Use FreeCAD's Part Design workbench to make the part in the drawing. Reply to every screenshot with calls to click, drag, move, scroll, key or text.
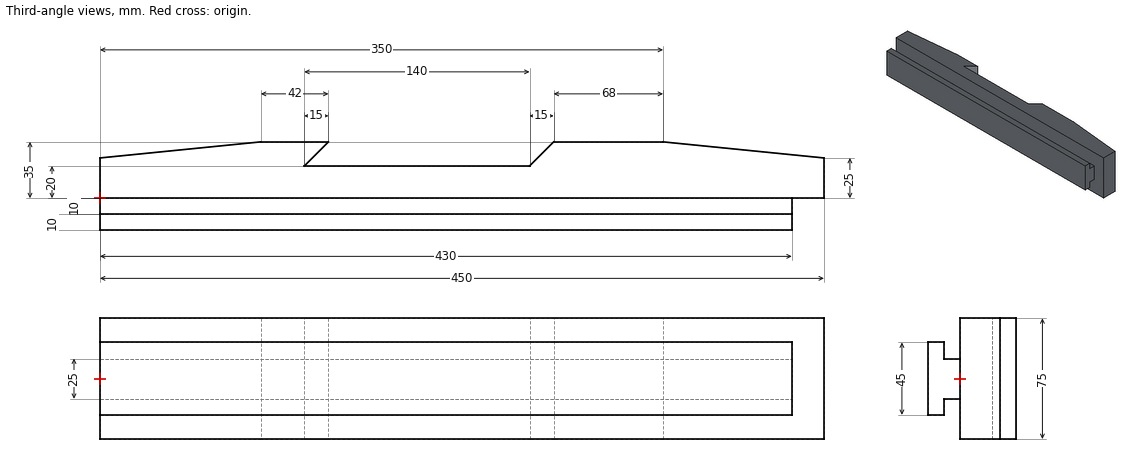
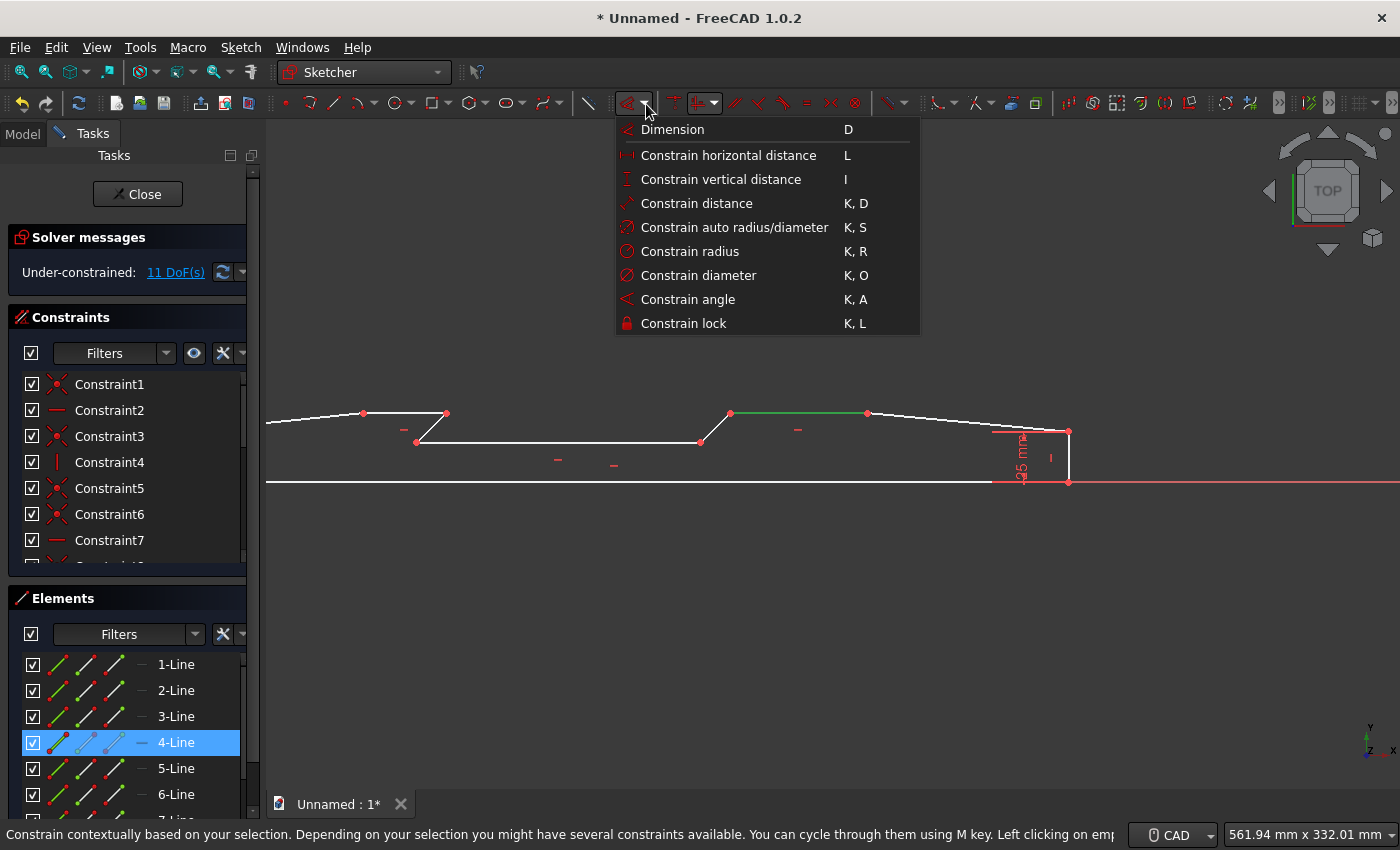
click(768, 155)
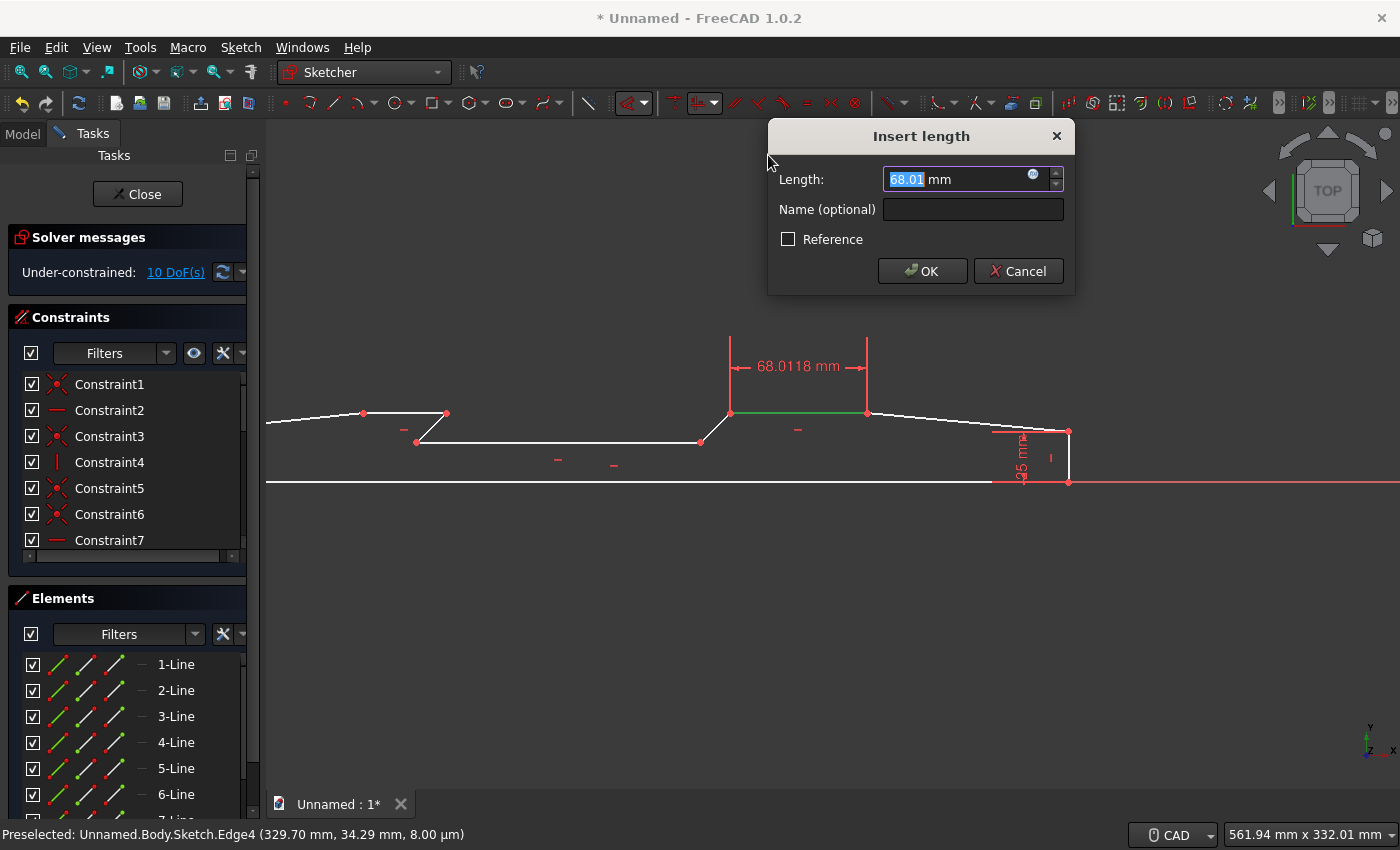
text(68)
key(Return)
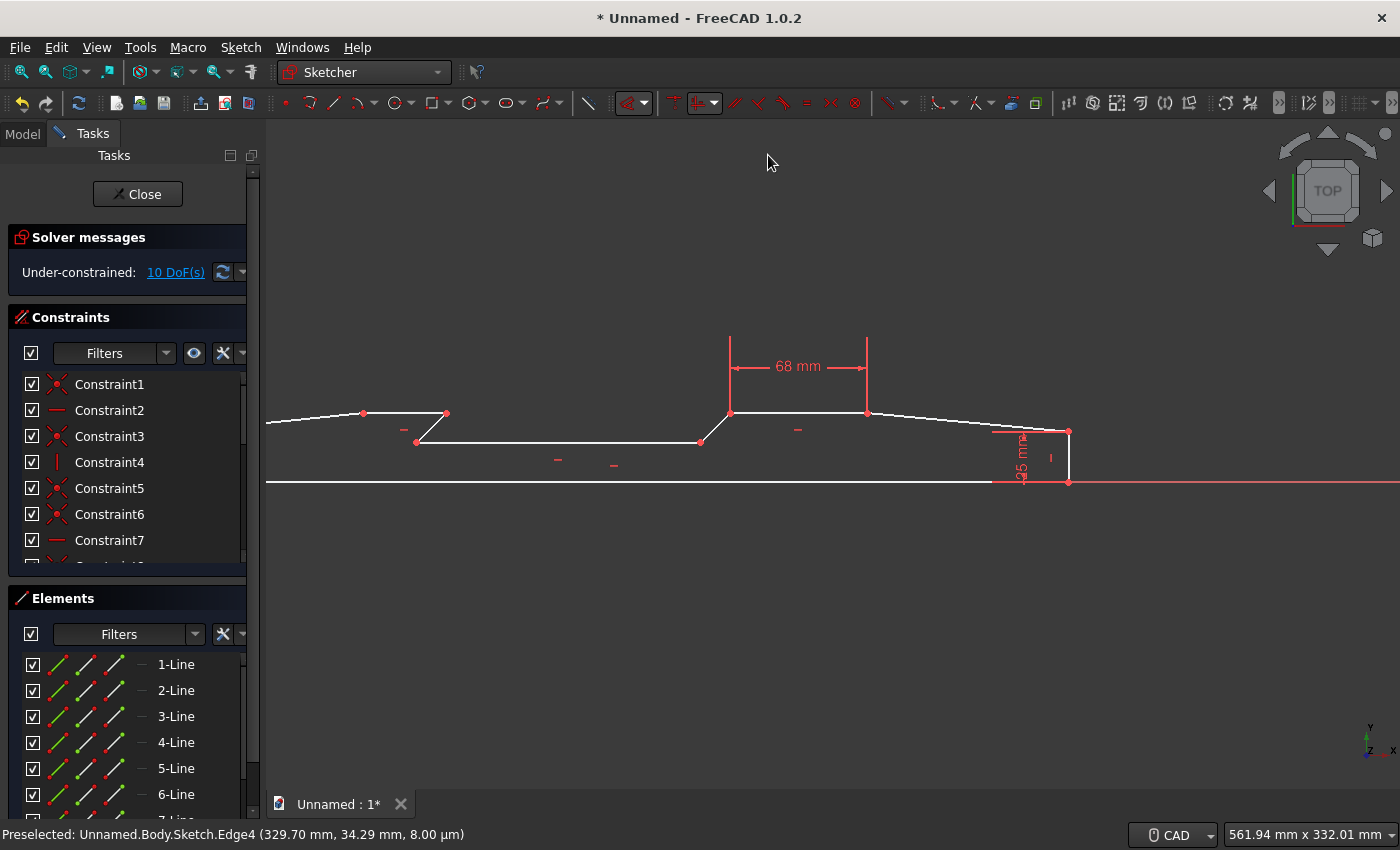
click(421, 413)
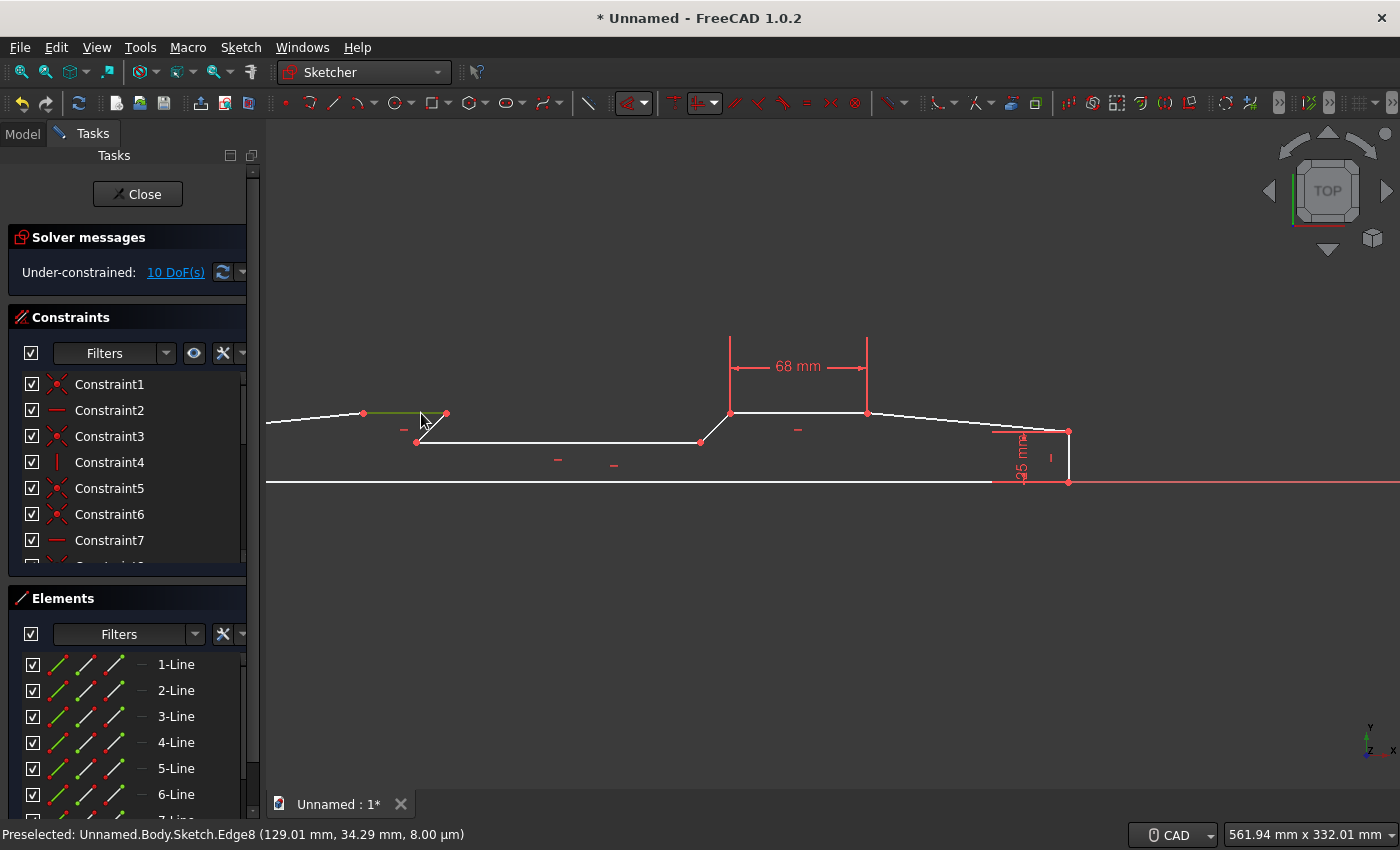
key(l)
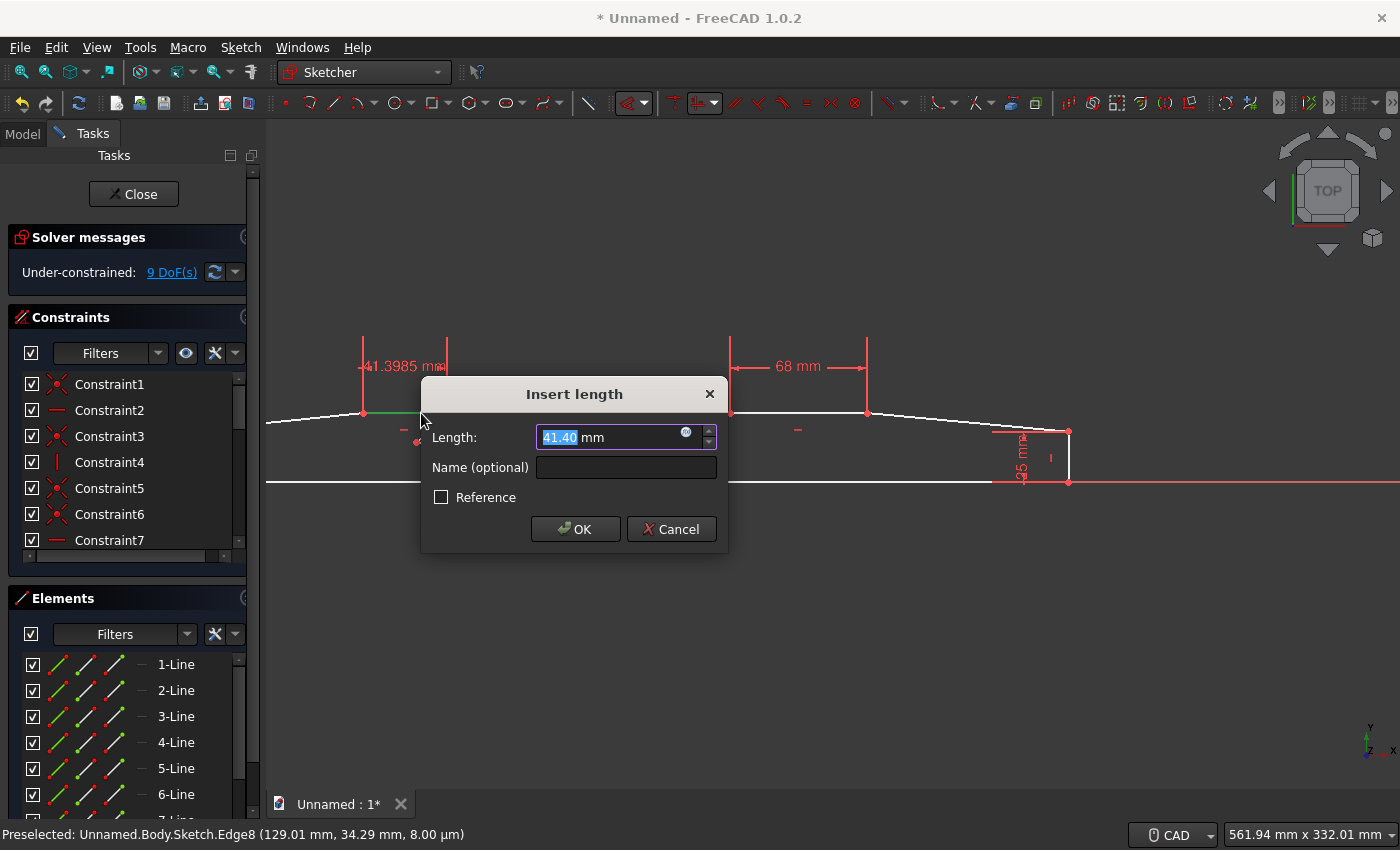
text(42)
key(Return)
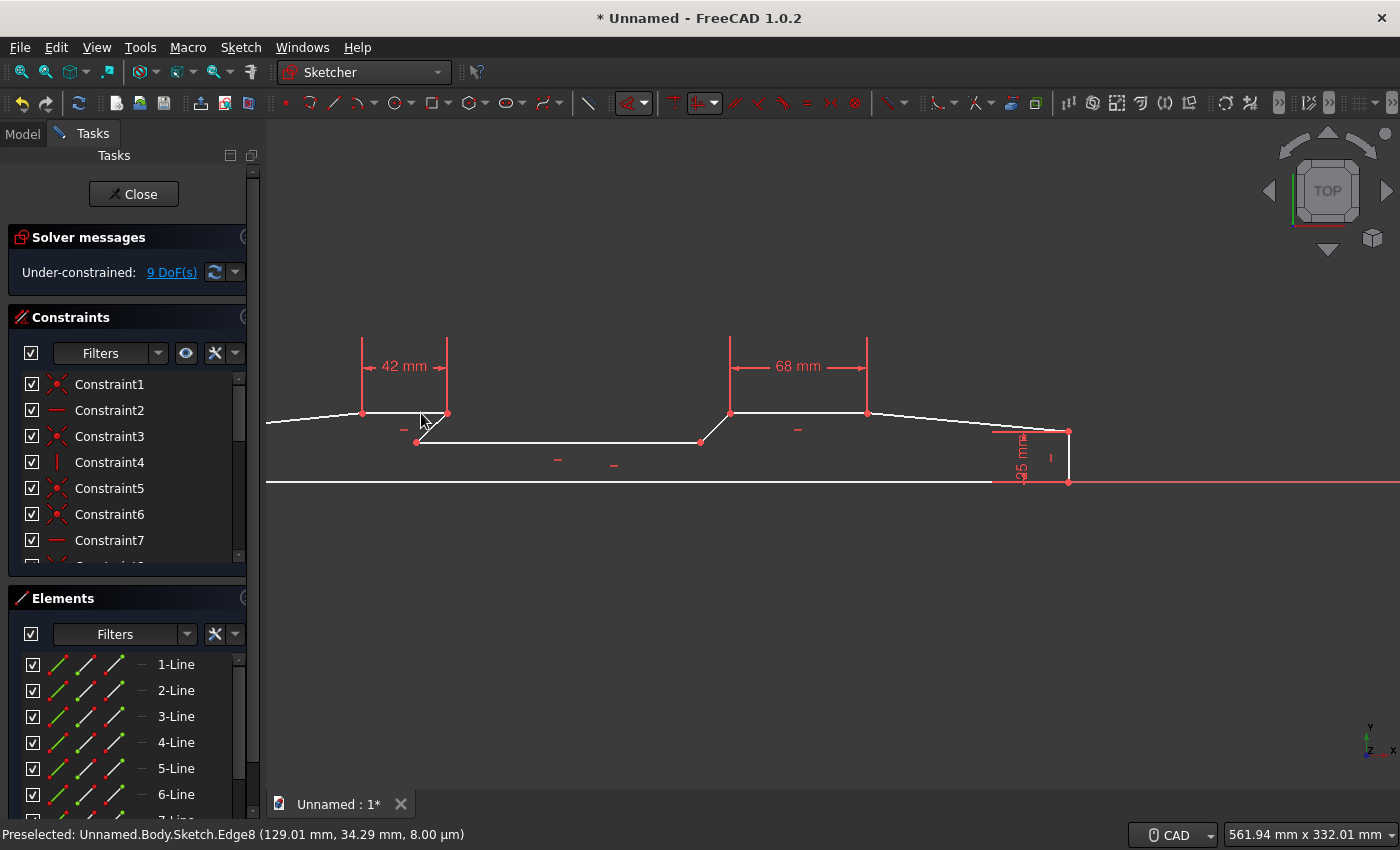
scroll(1069, 468, down, 2)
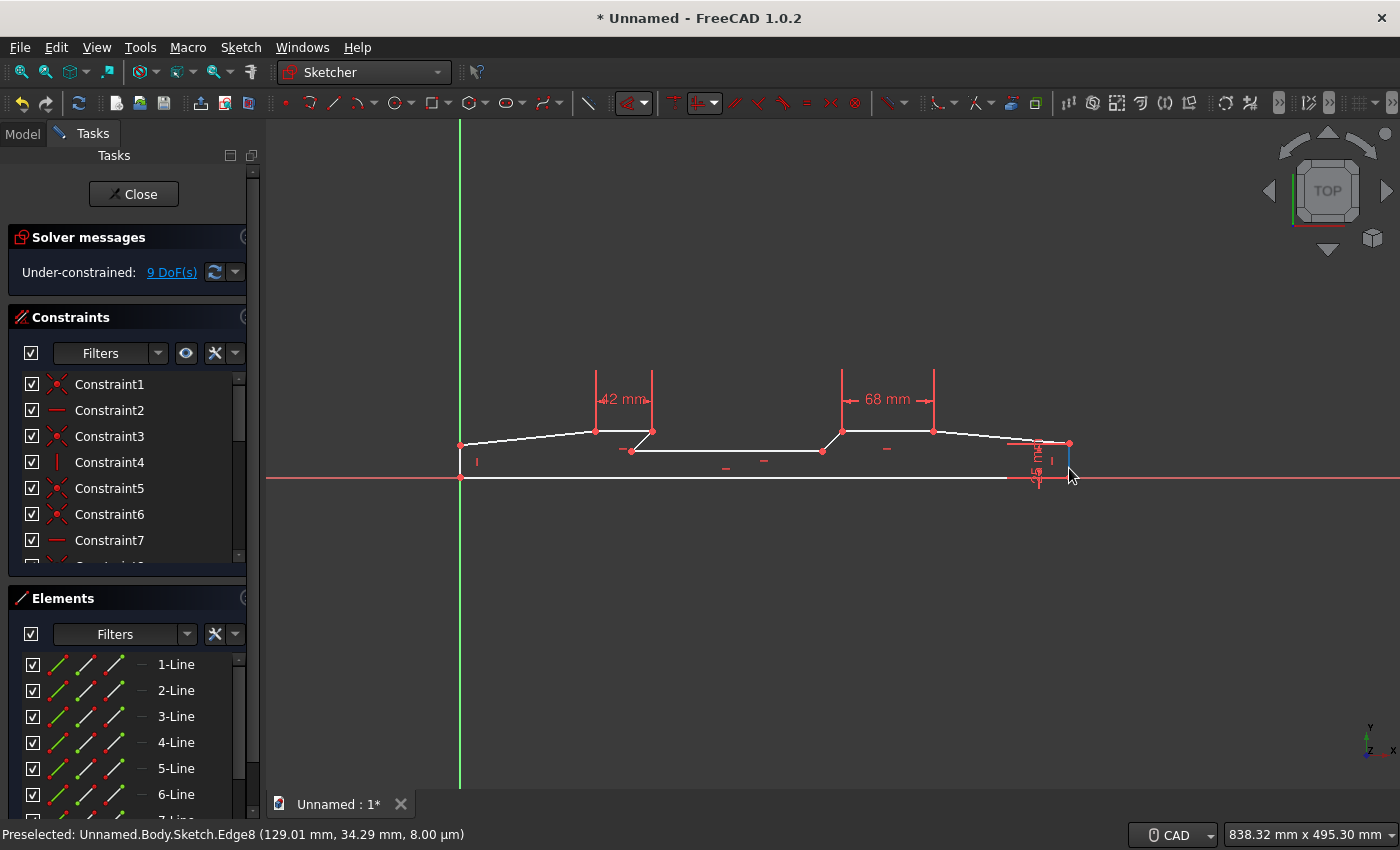
scroll(460, 455, up, 2)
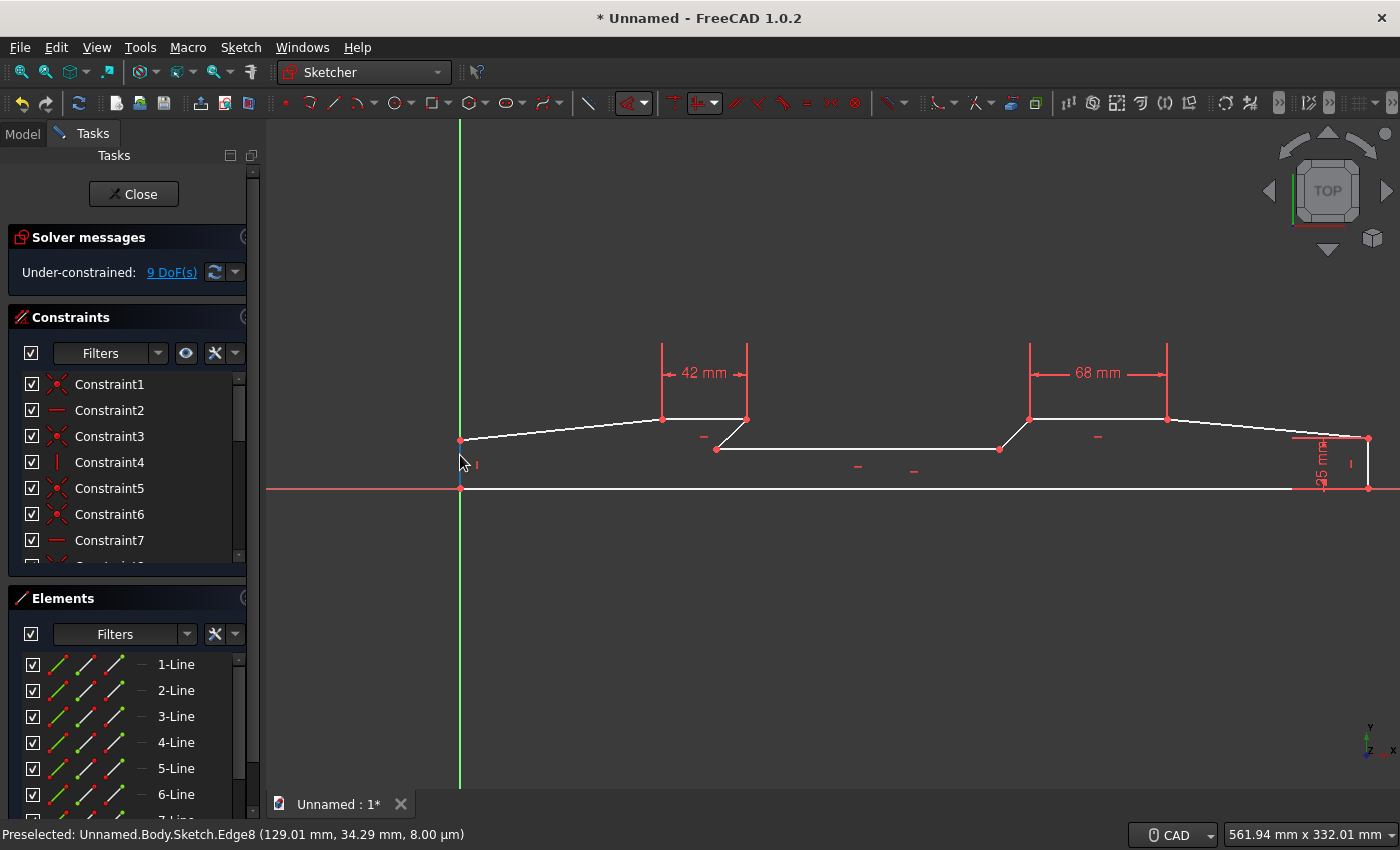
click(460, 455)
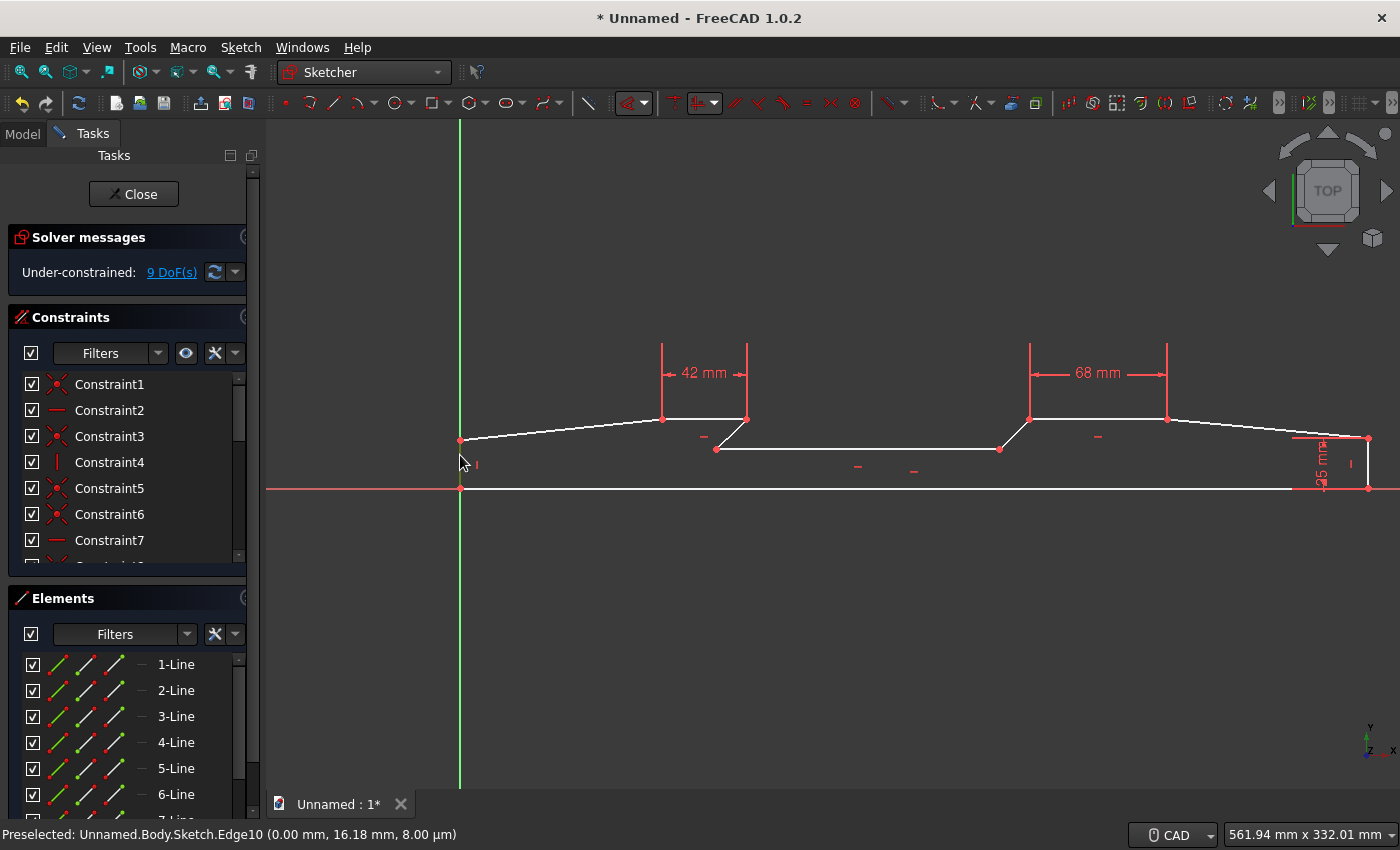
key(i)